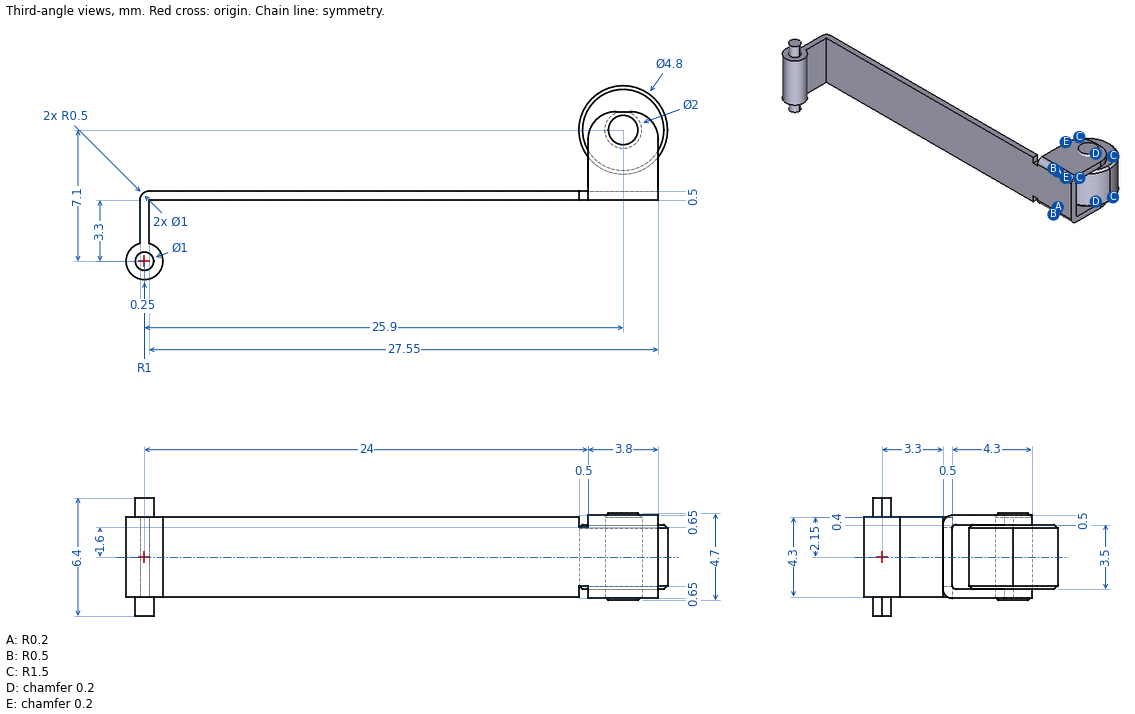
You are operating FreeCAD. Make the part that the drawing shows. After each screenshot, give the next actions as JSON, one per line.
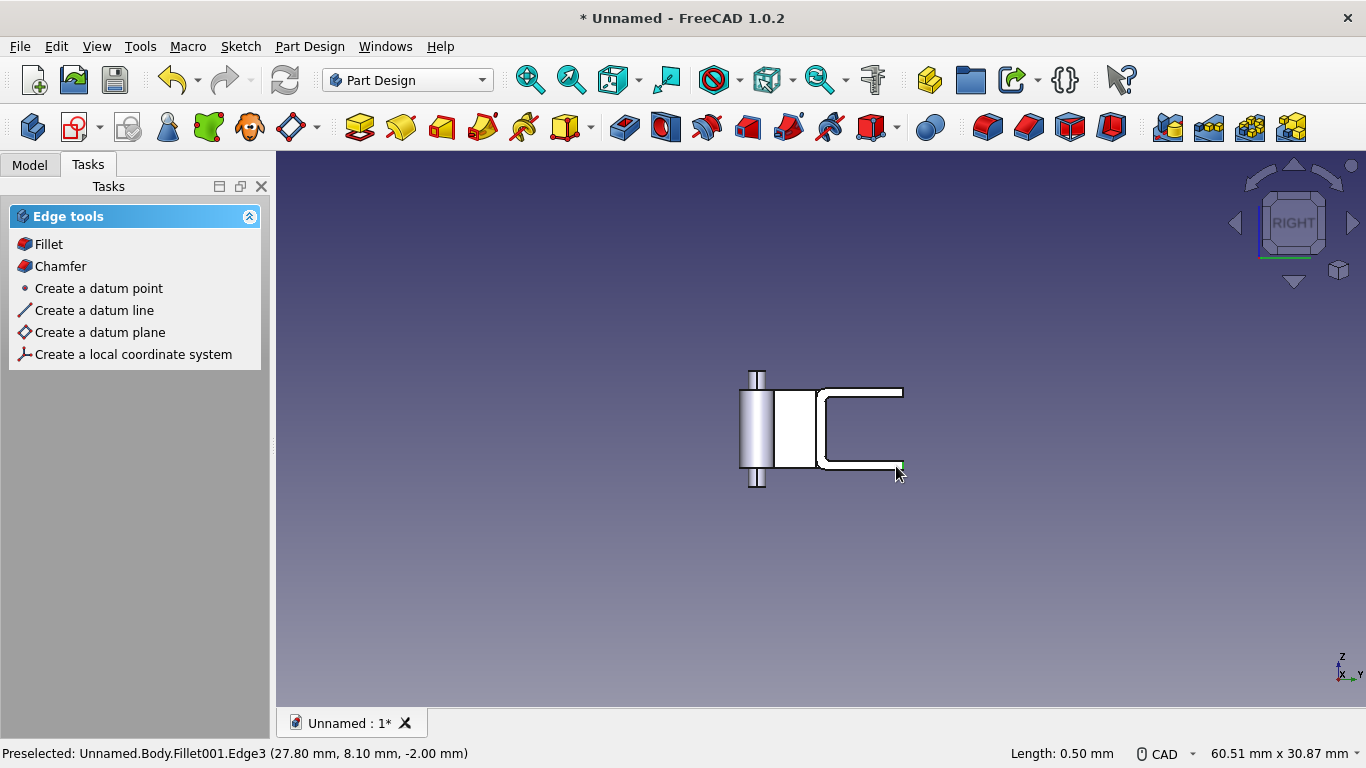
{"action": "key", "text": "5"}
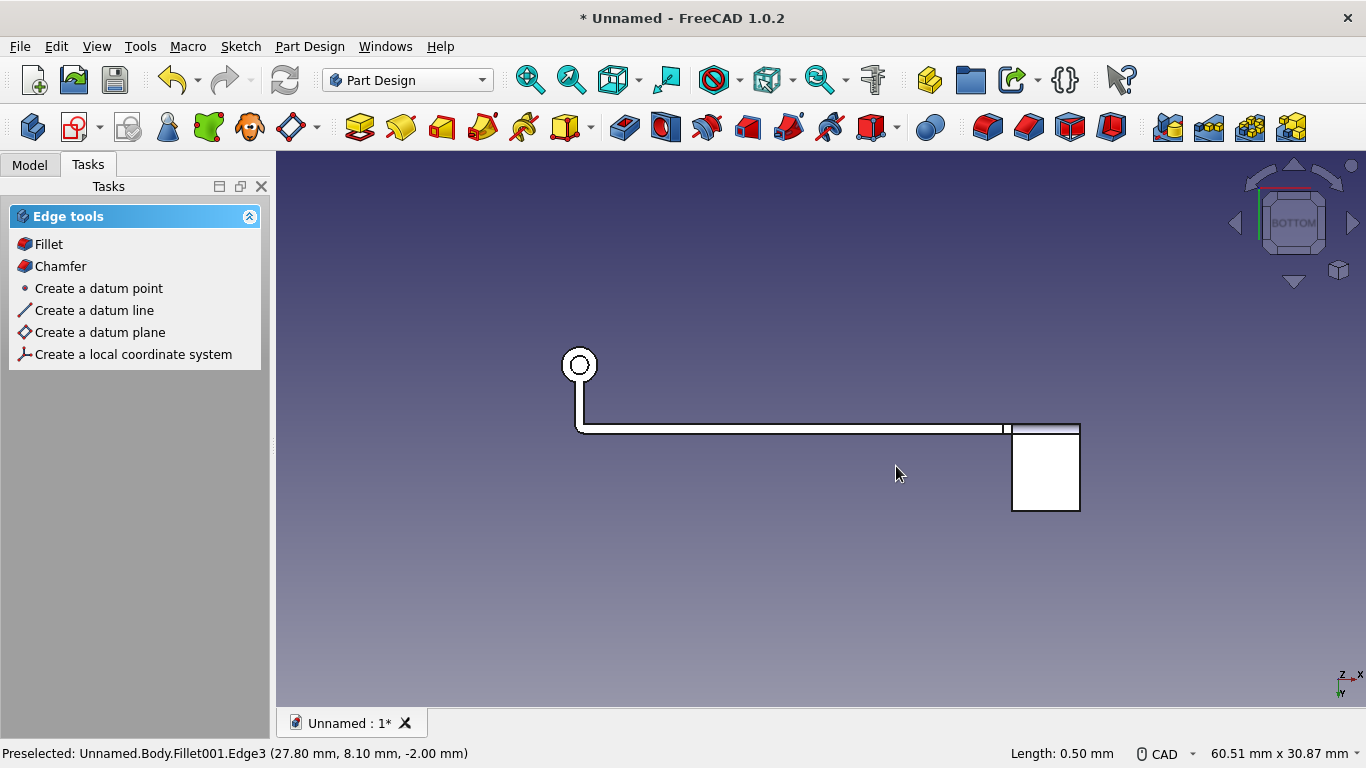
{"action": "scroll", "coordinate": [1012, 510], "scroll_direction": "up", "scroll_amount": 8}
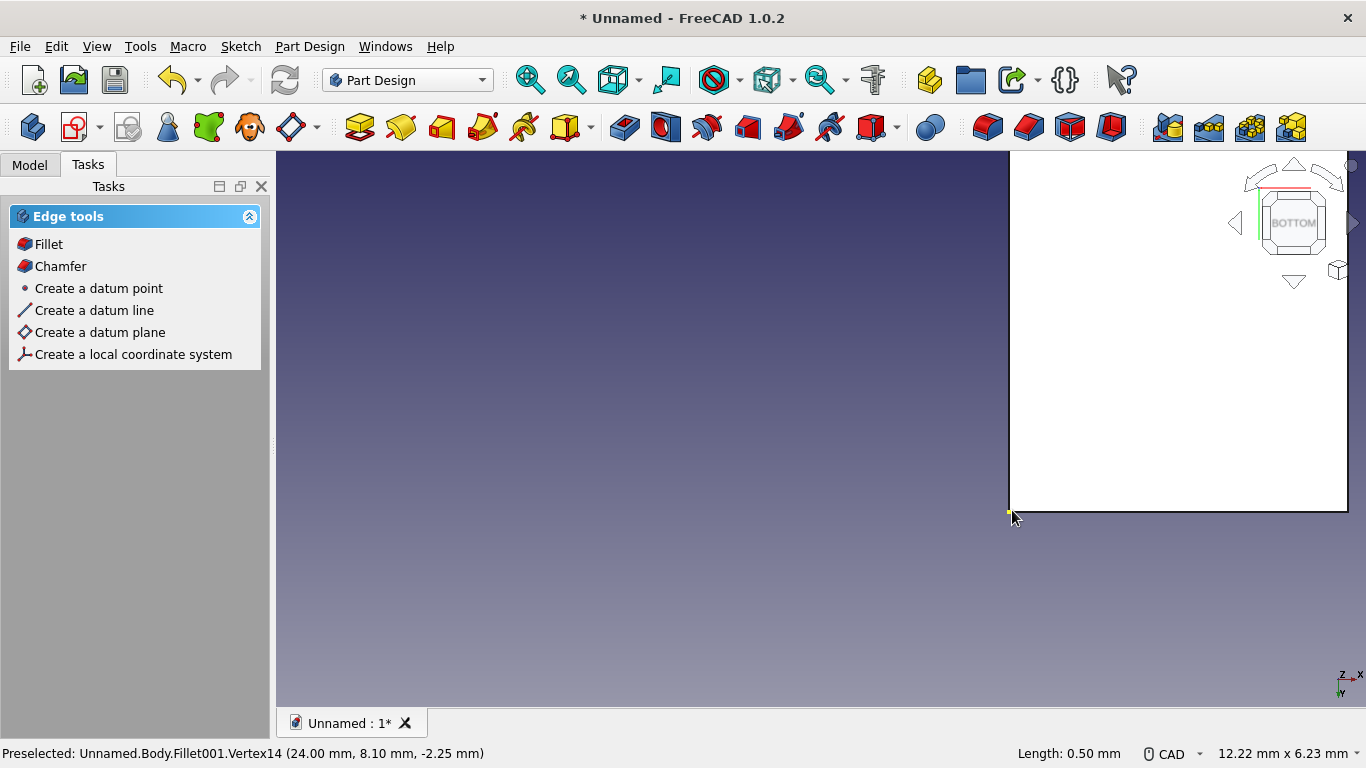
{"action": "key", "text": "v f"}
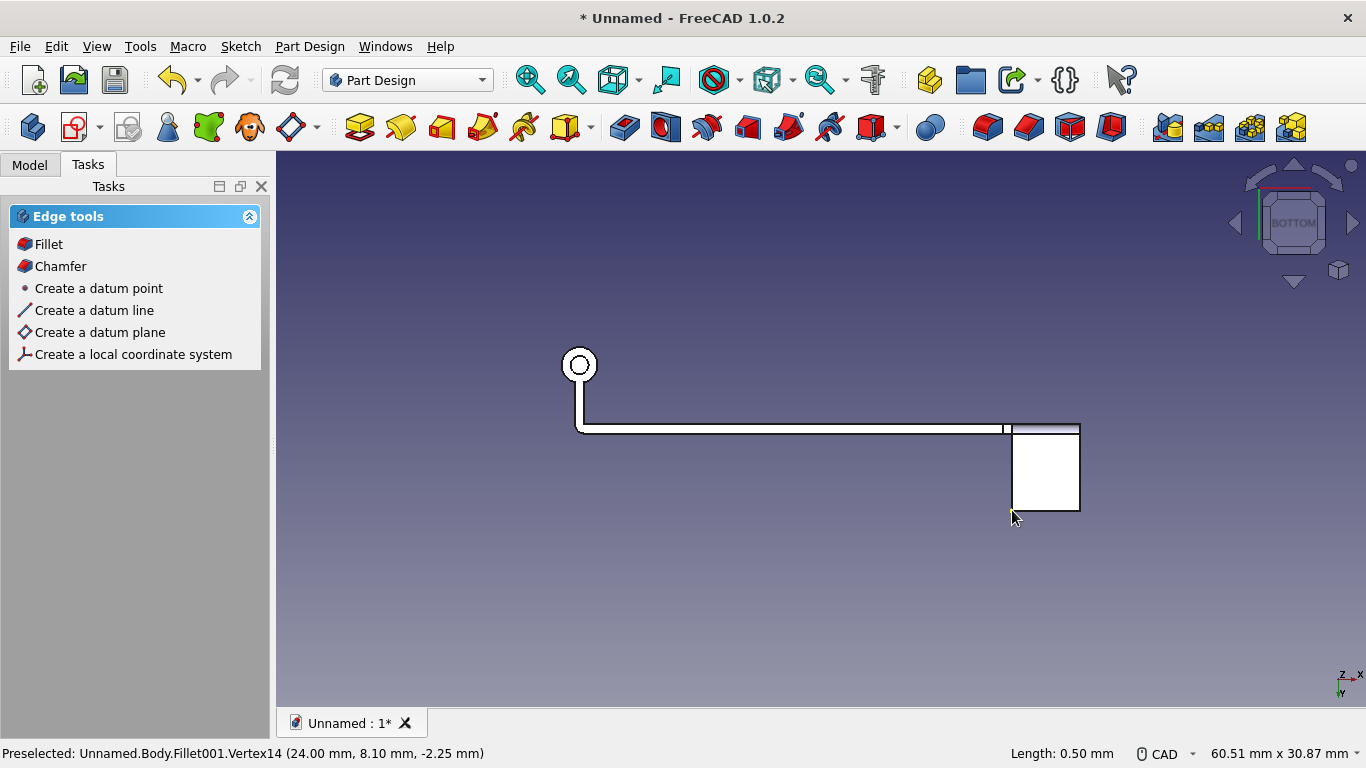
{"action": "key", "text": "4"}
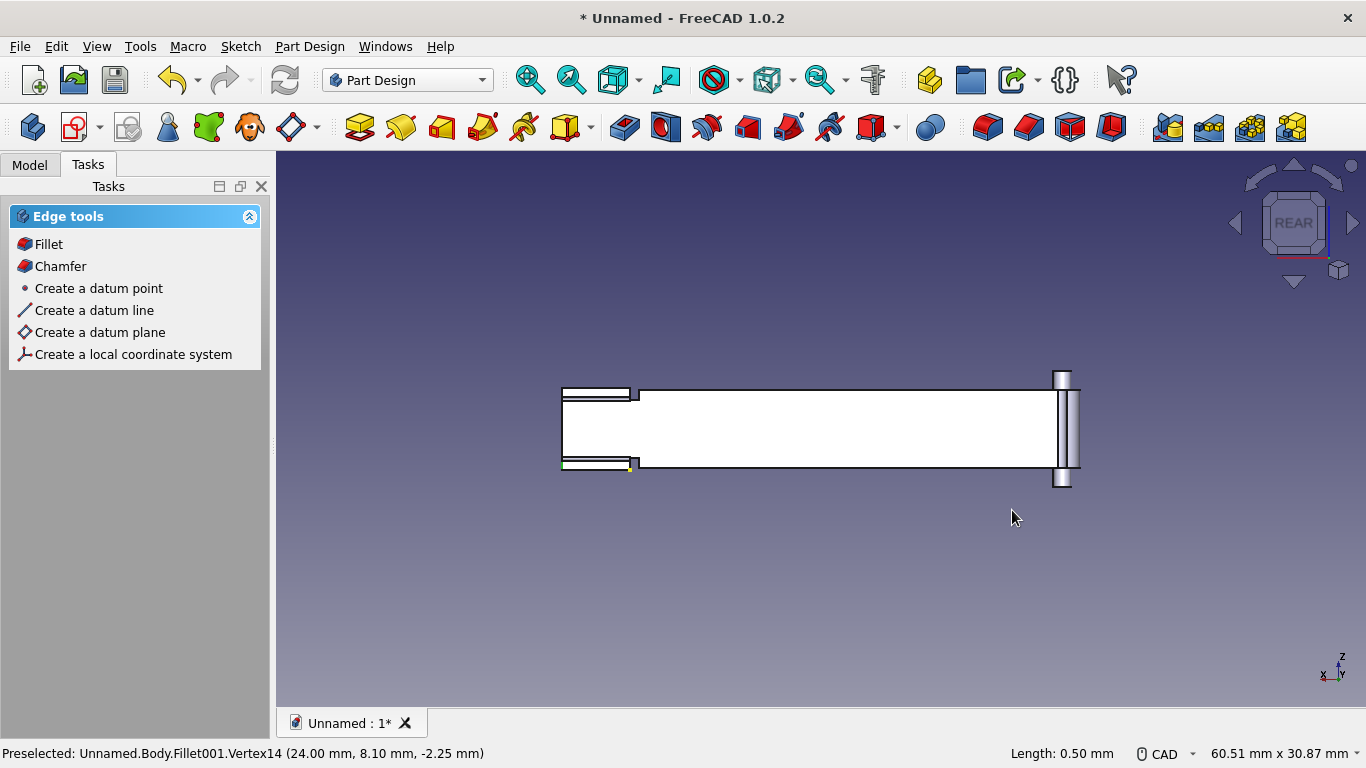
{"action": "scroll", "coordinate": [630, 464], "scroll_direction": "up", "scroll_amount": 8}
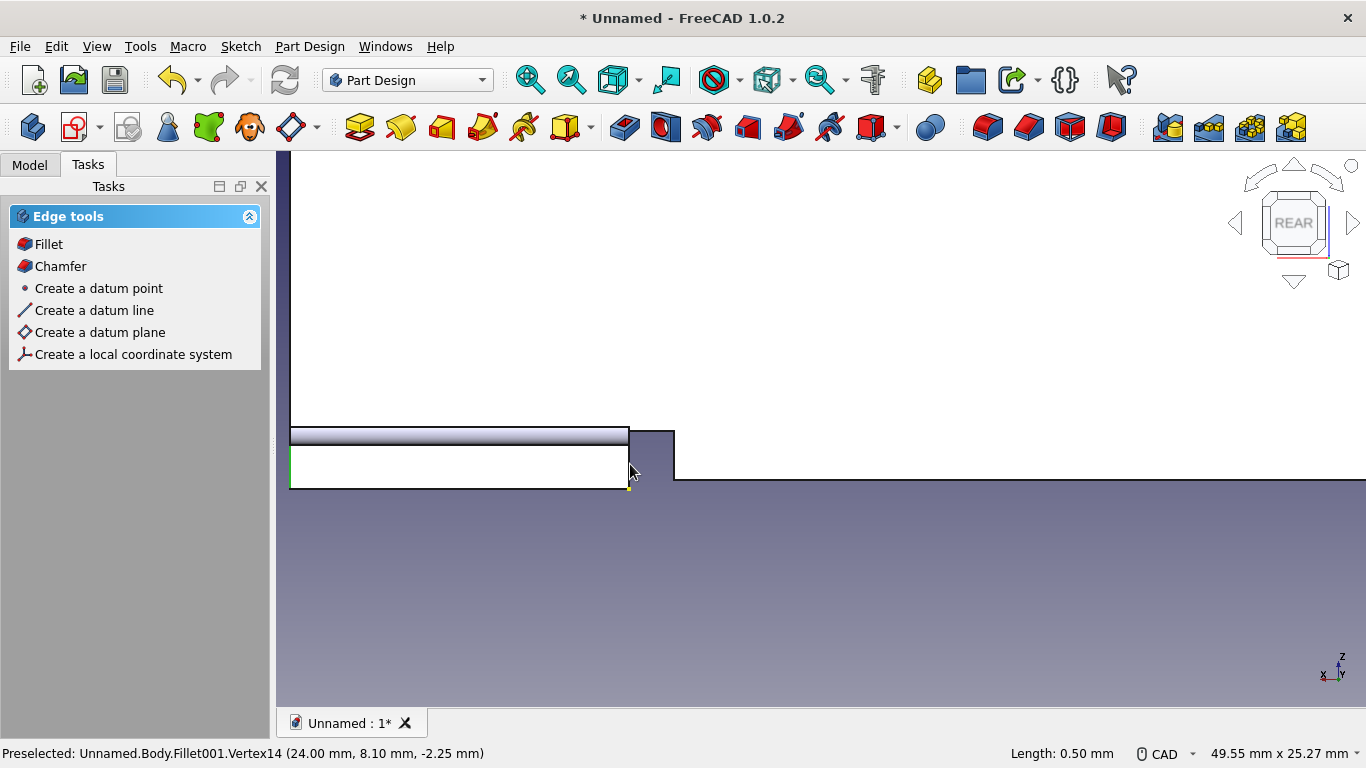
{"action": "left_click", "coordinate": [629, 466], "text": "ctrl"}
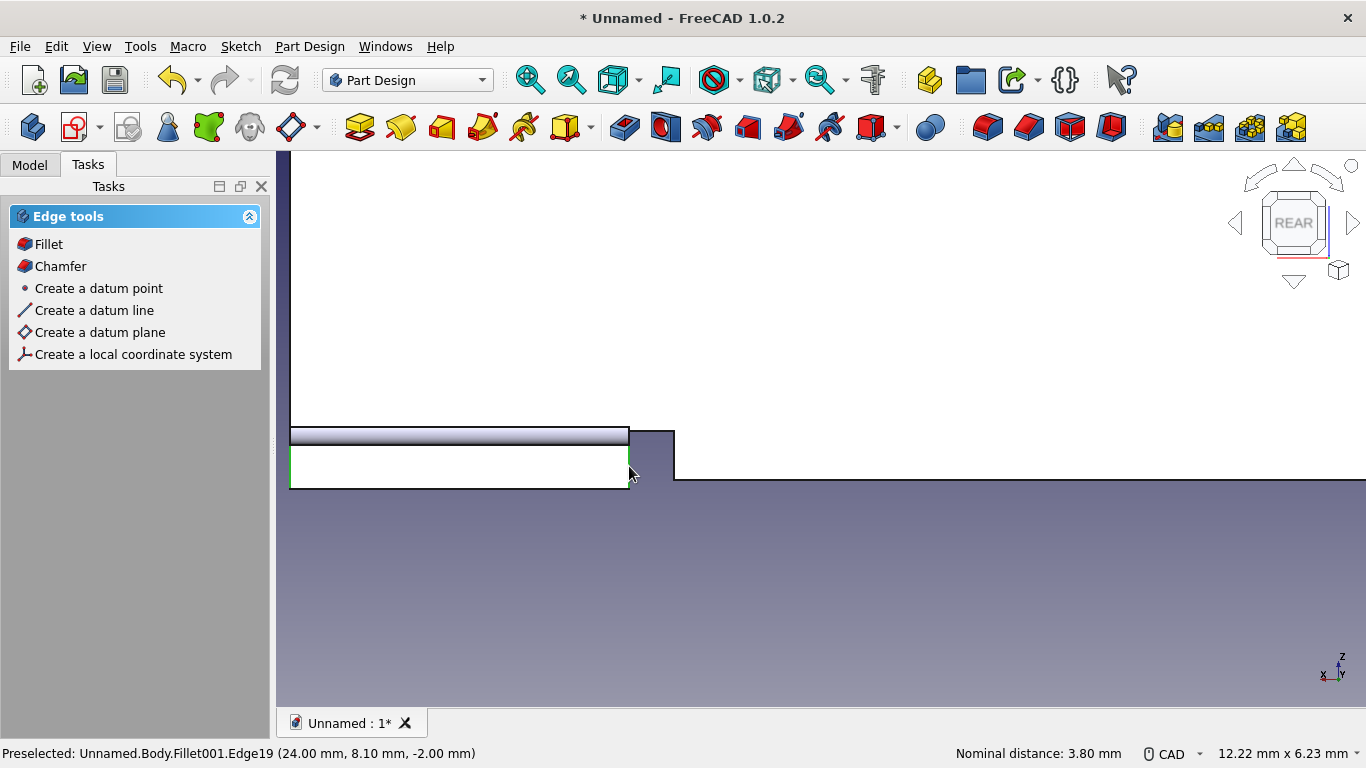
{"action": "left_click", "coordinate": [531, 80]}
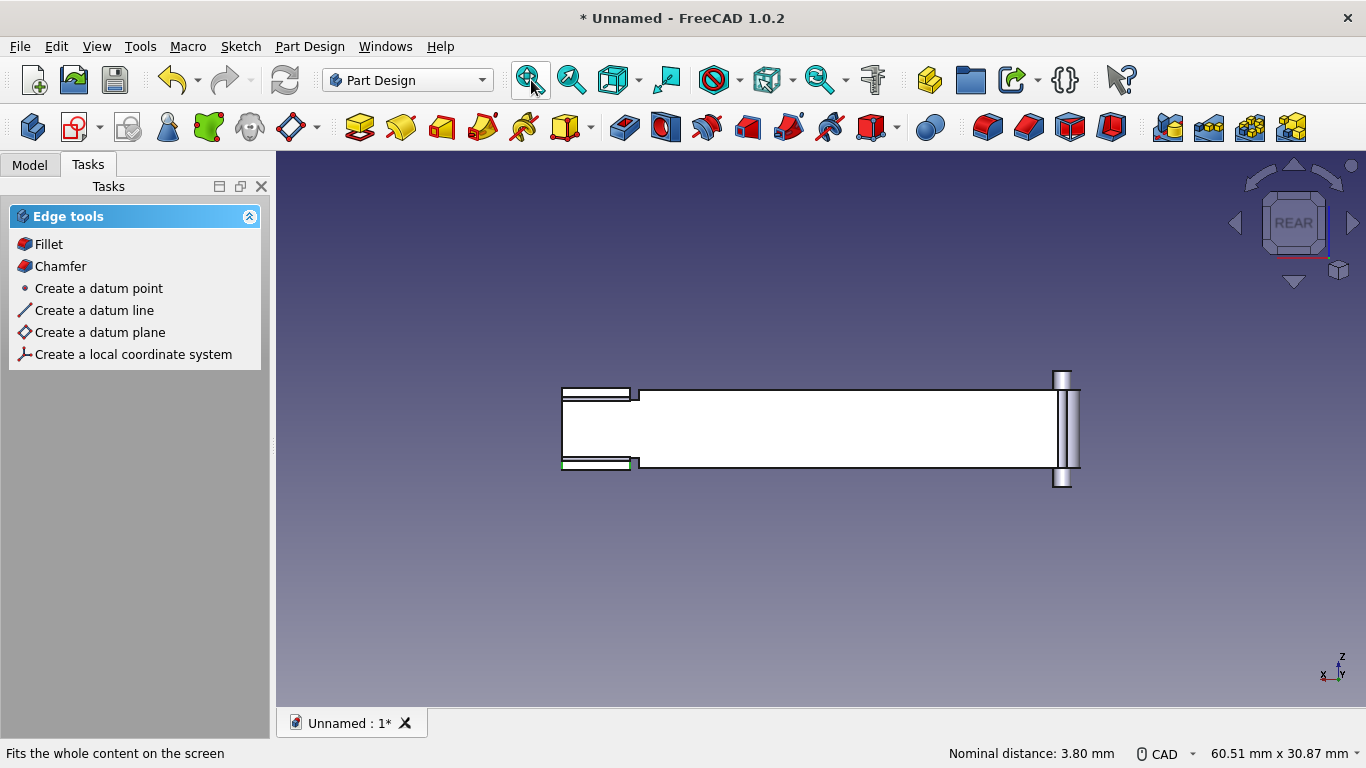
{"action": "key", "text": "6"}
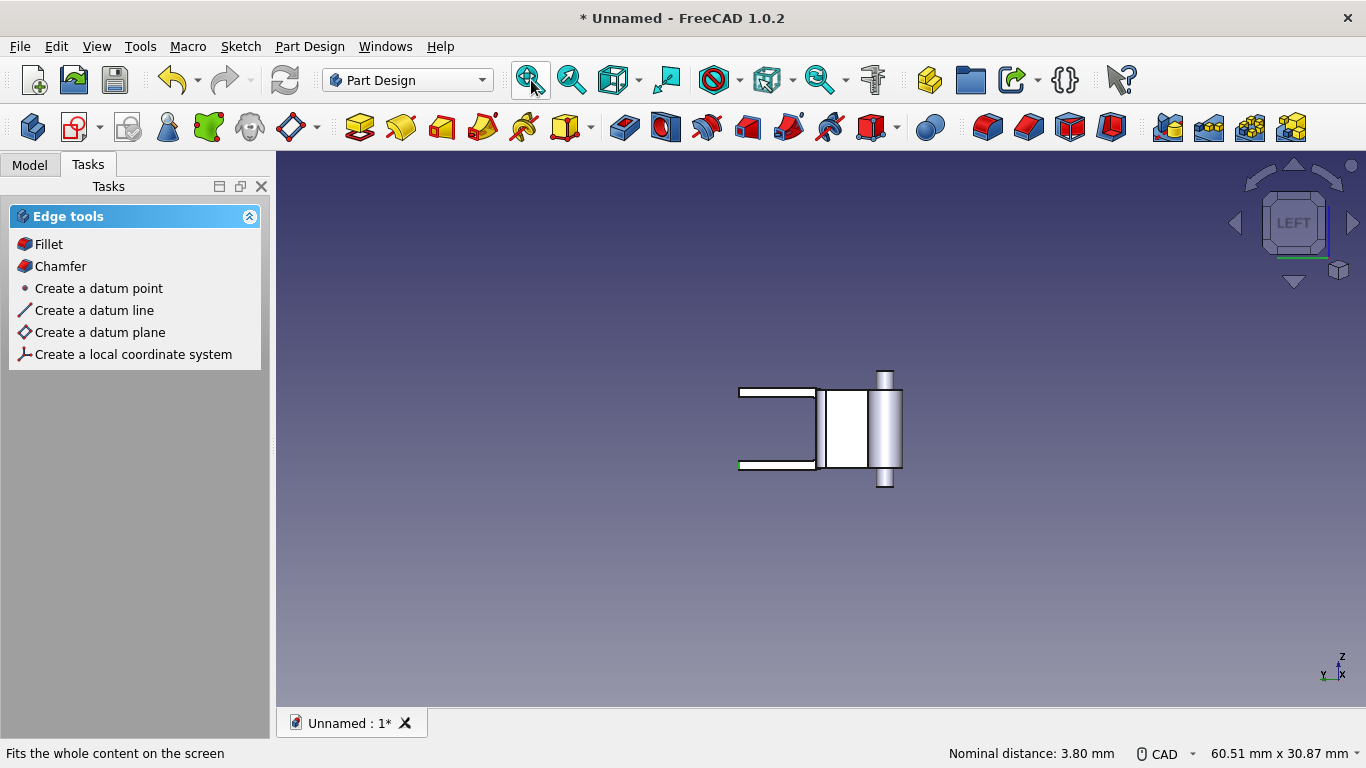
{"action": "key", "text": "v f"}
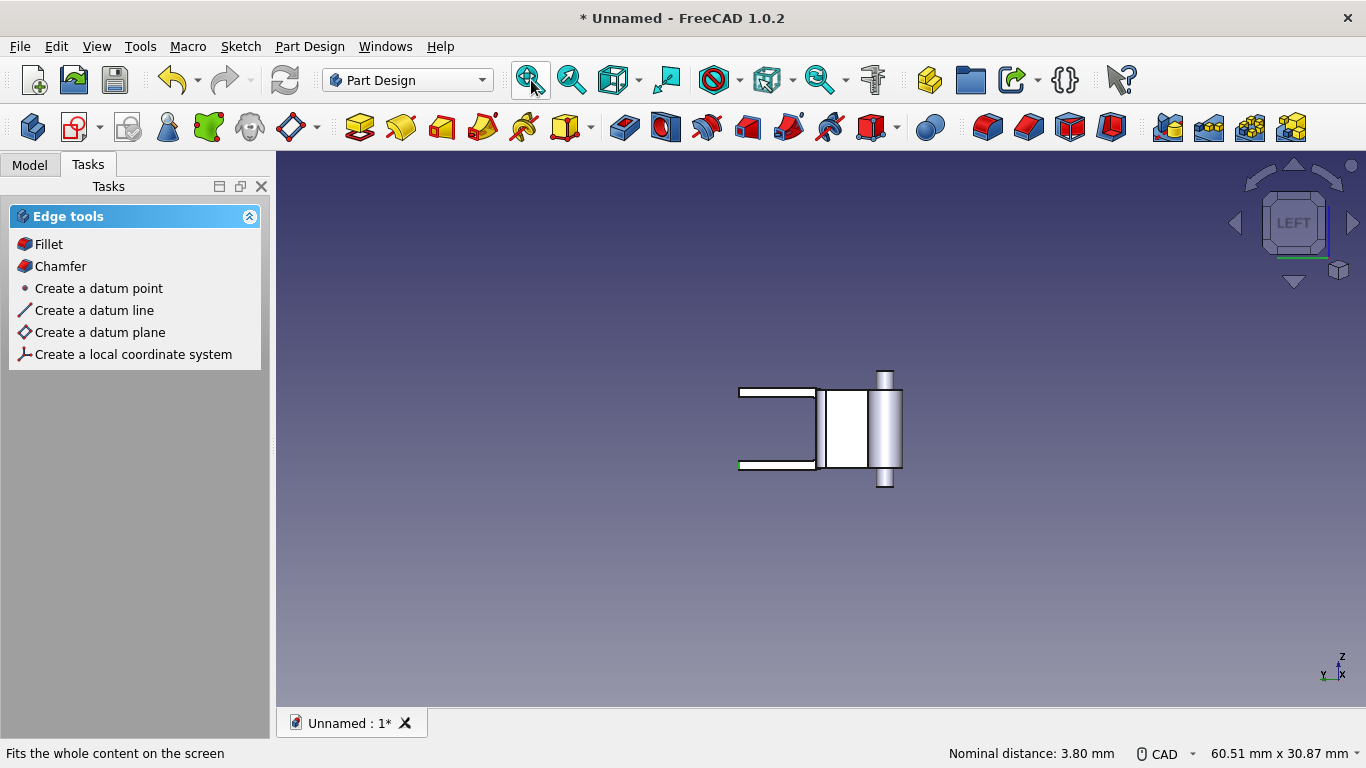
{"action": "scroll", "coordinate": [739, 392], "scroll_direction": "up", "scroll_amount": 8}